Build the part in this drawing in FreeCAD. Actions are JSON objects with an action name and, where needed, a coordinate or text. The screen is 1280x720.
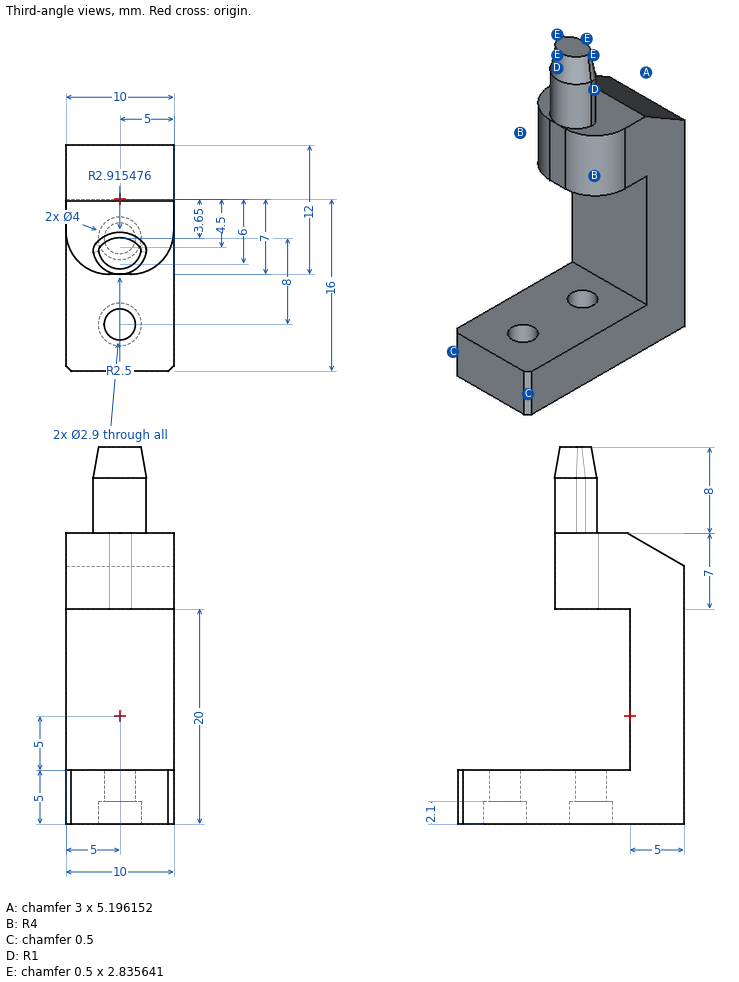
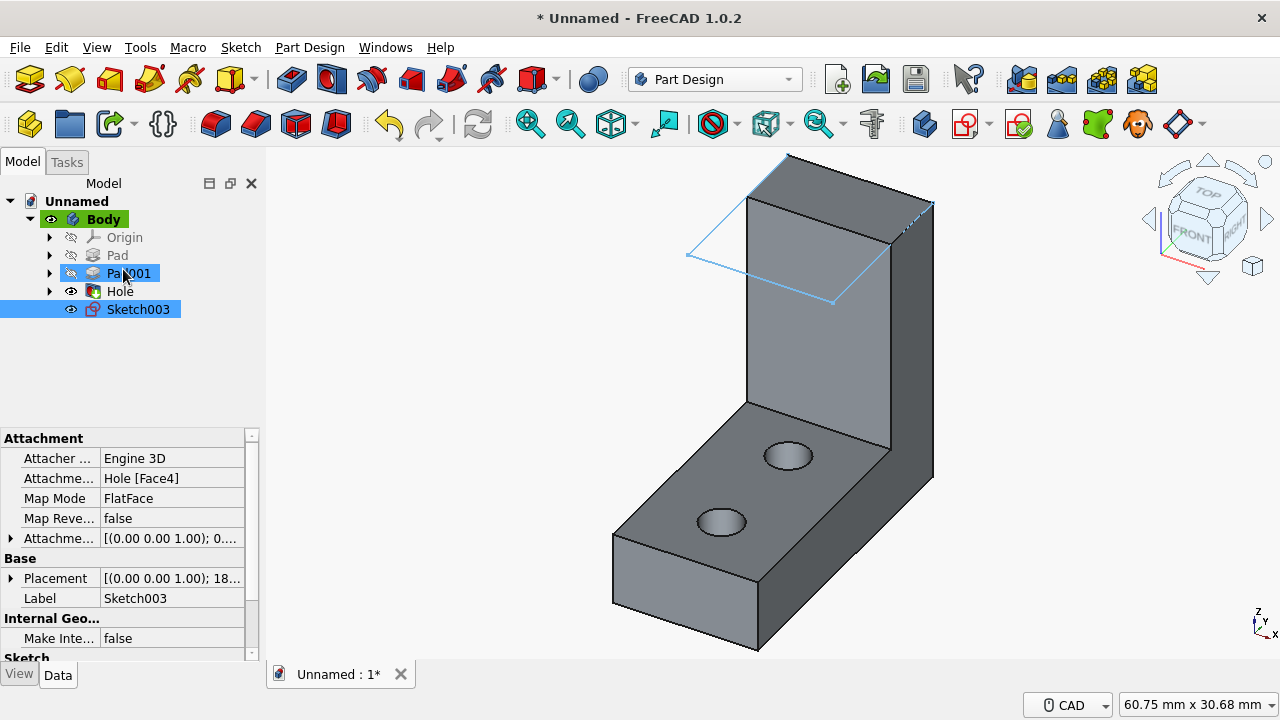
{"action": "left_click", "coordinate": [30, 80]}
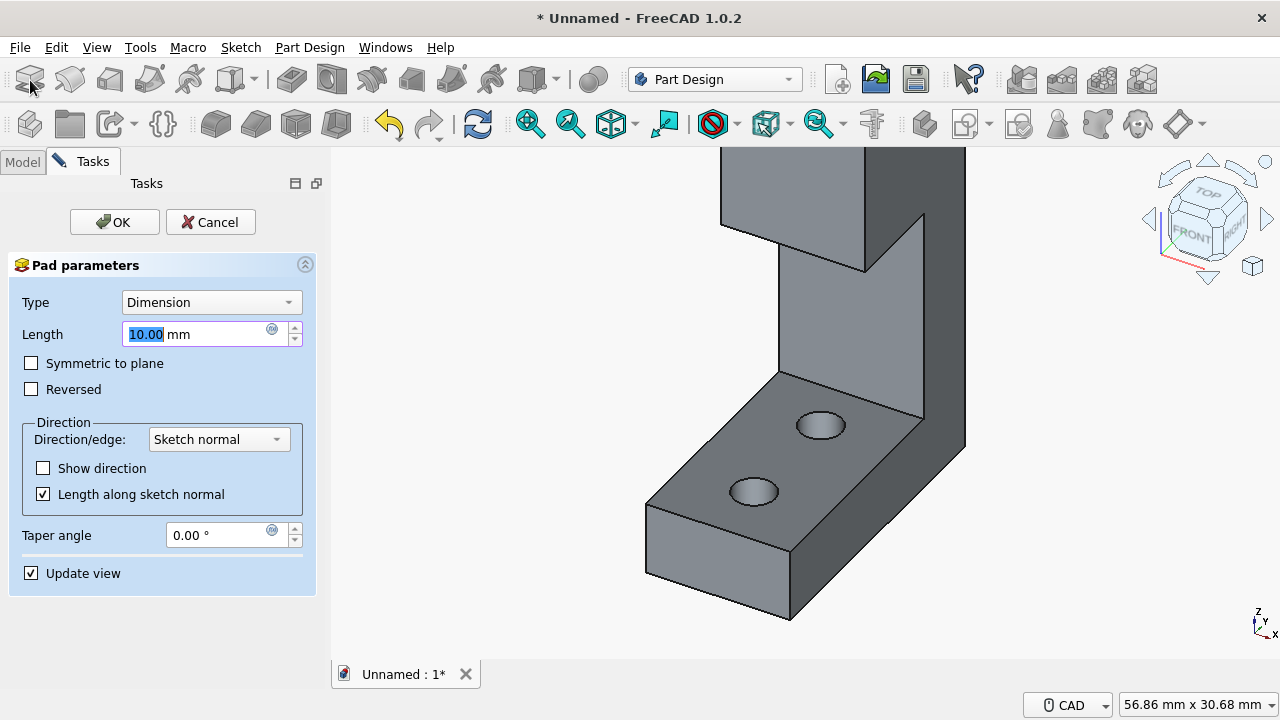
{"action": "type", "text": "7"}
{"action": "key", "text": "Tab"}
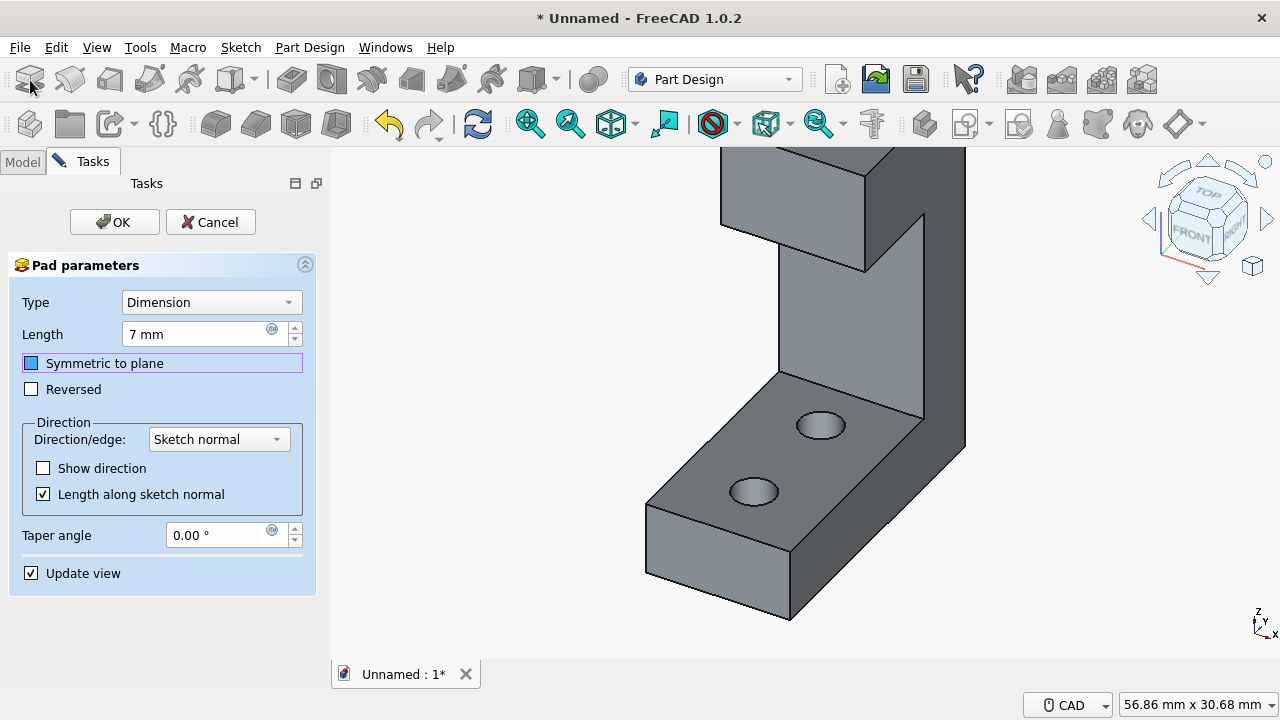
{"action": "left_click", "coordinate": [115, 222]}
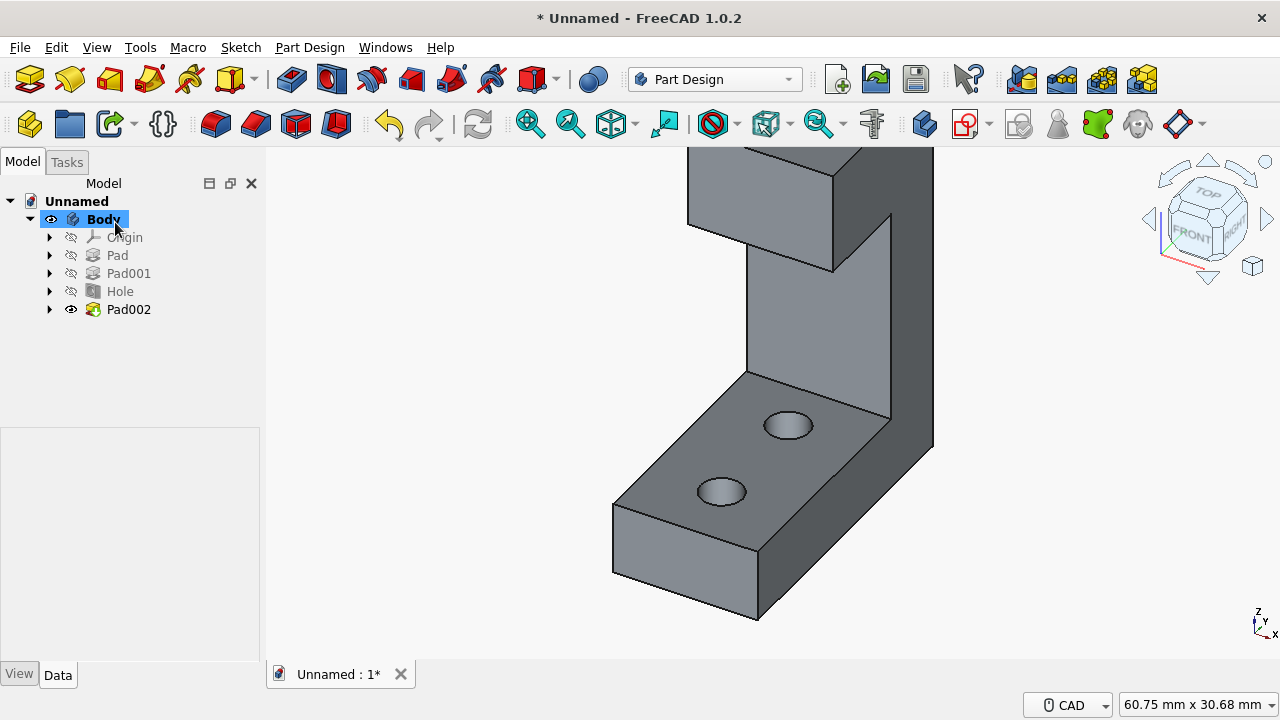
{"action": "left_click", "coordinate": [532, 124]}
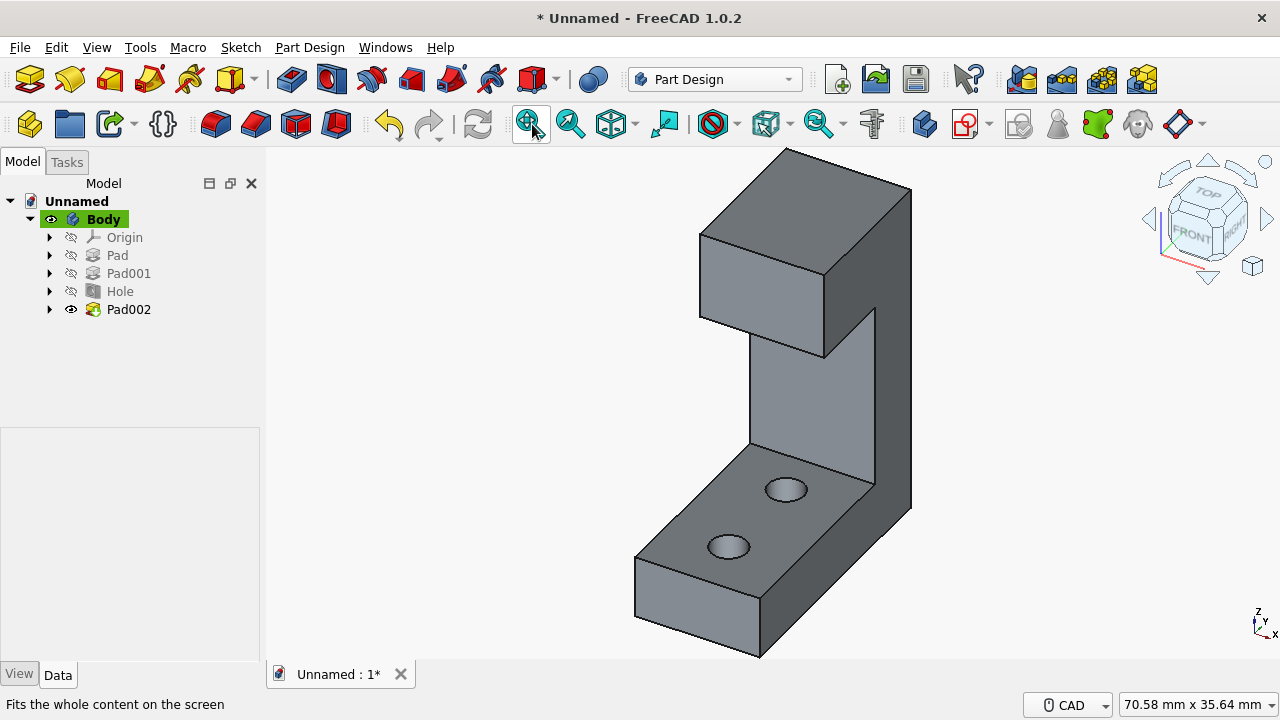
{"action": "key", "text": "0"}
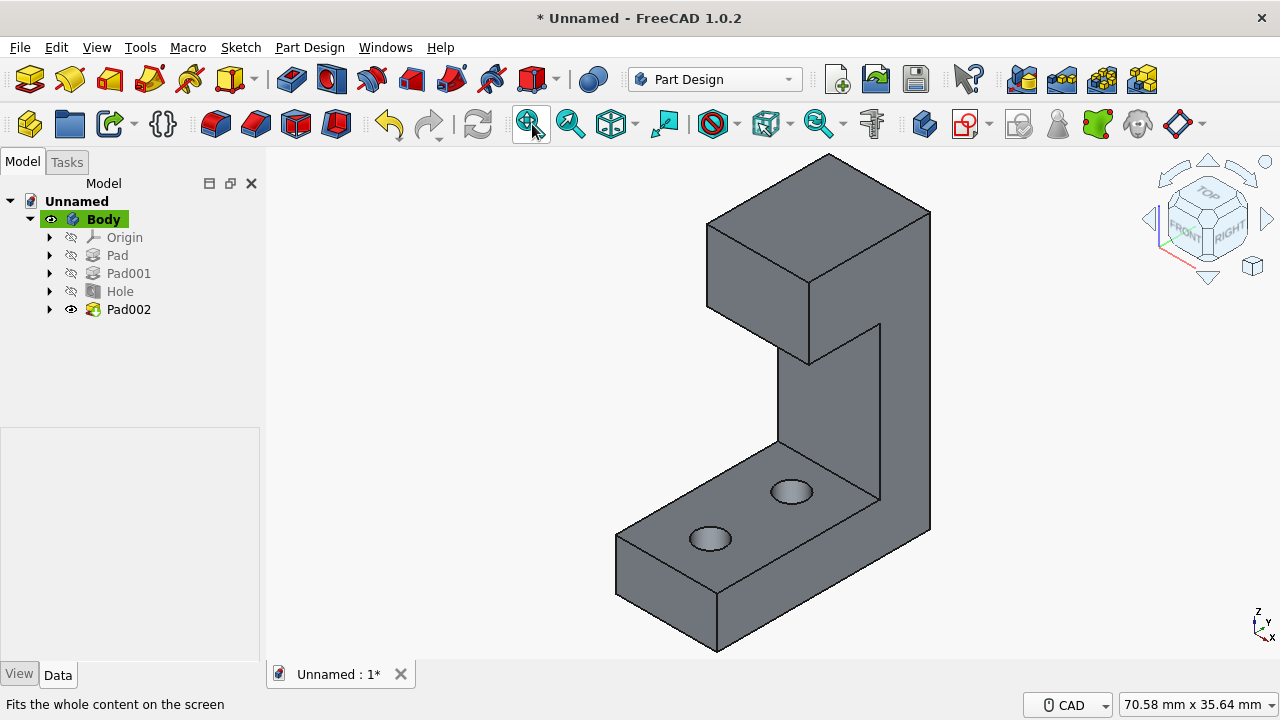
{"action": "key", "text": "2"}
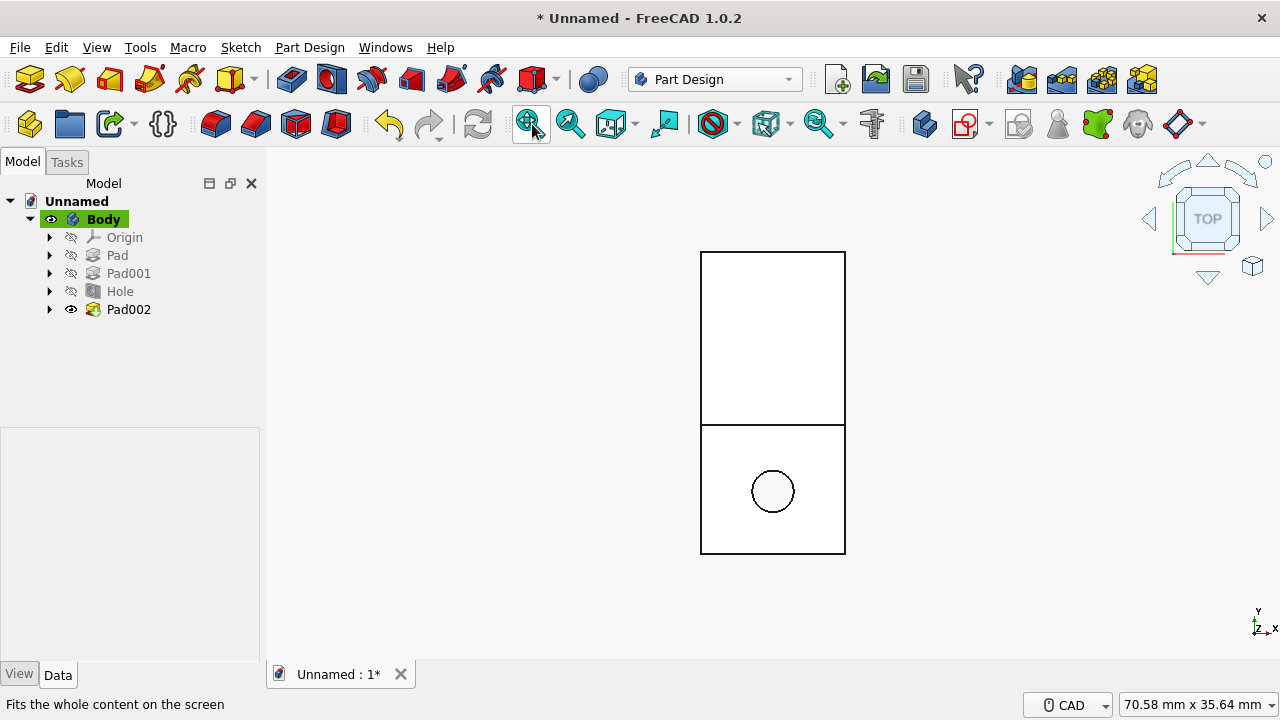
{"action": "left_click", "coordinate": [773, 251]}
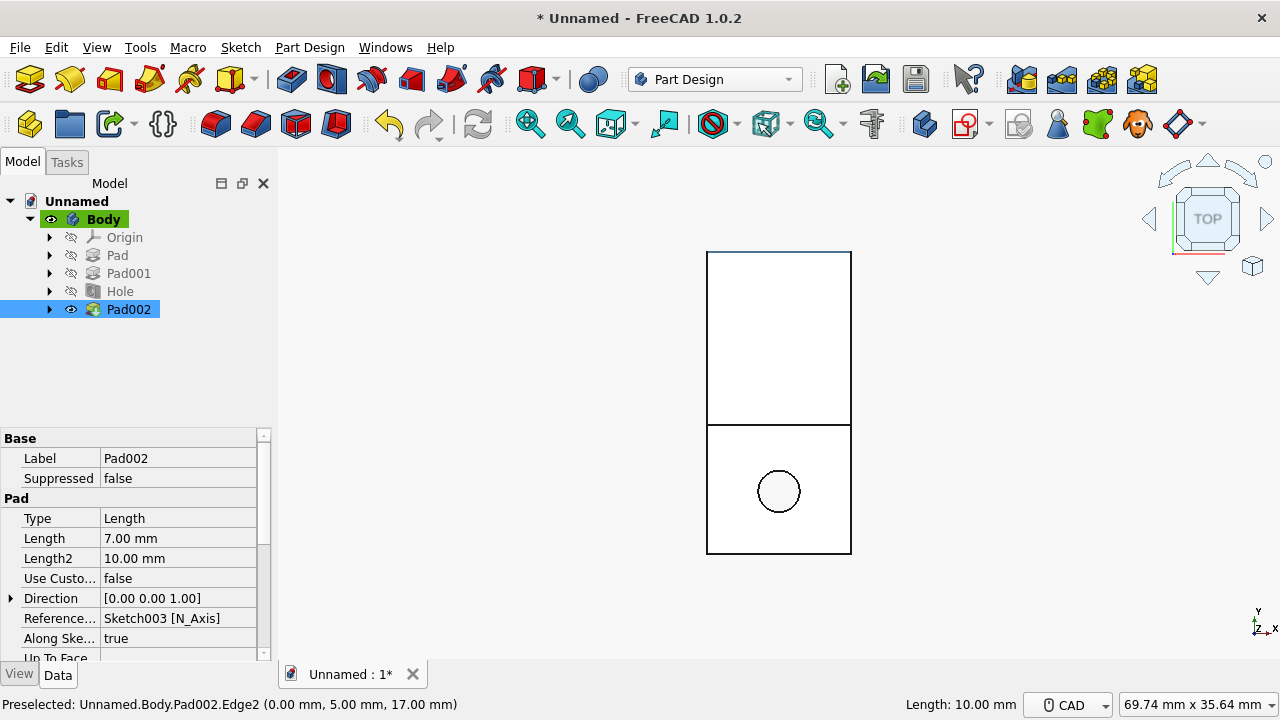
{"action": "left_click", "coordinate": [256, 124]}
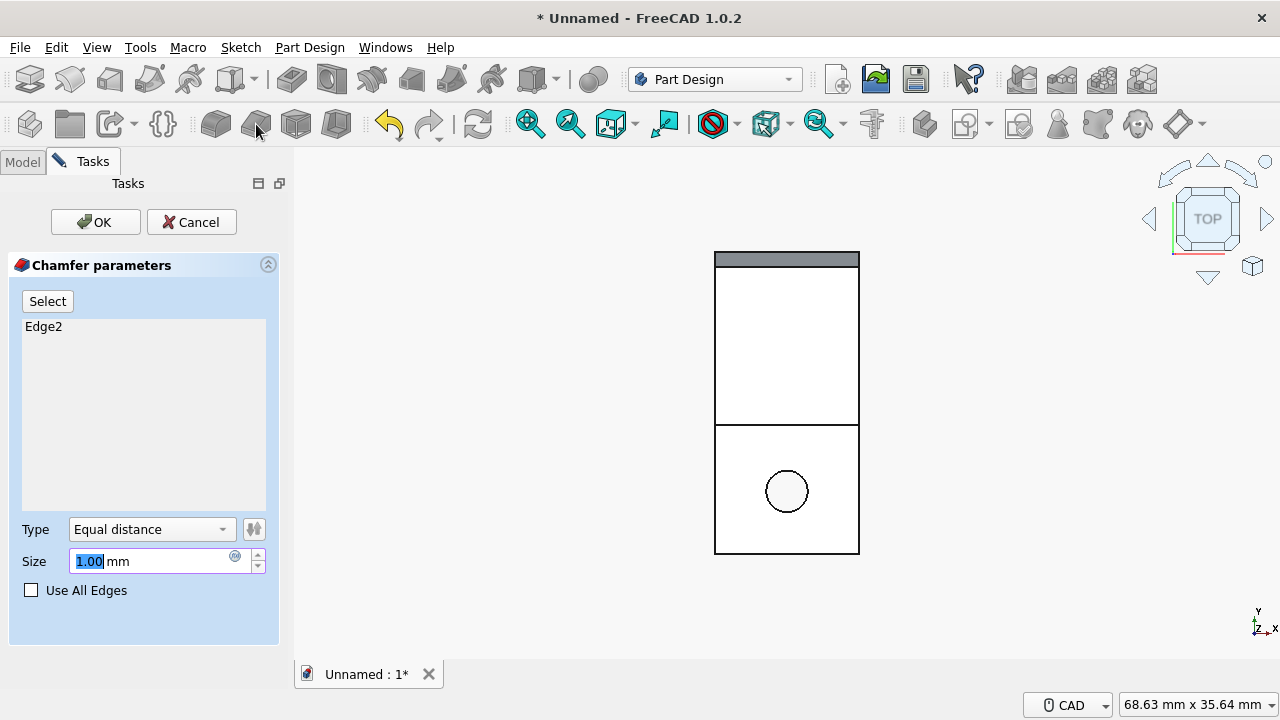
{"action": "type", "text": "3"}
{"action": "key", "text": "Tab"}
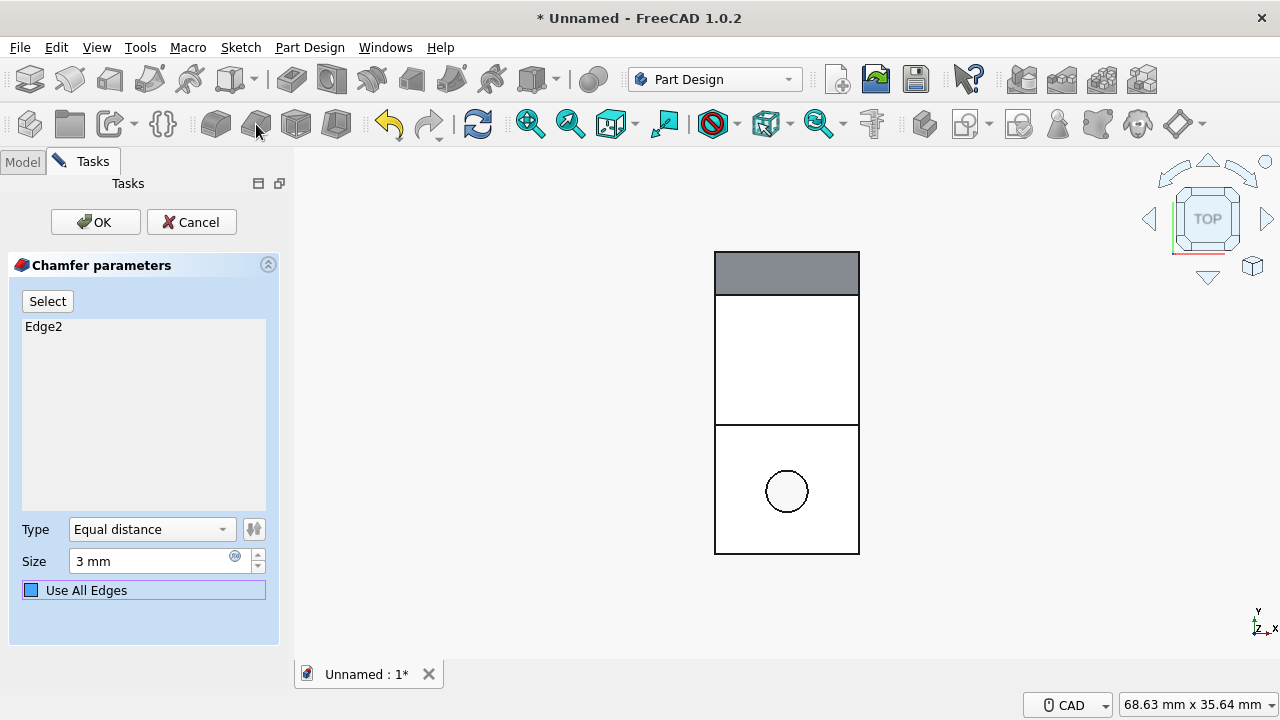
{"action": "left_click", "coordinate": [153, 530]}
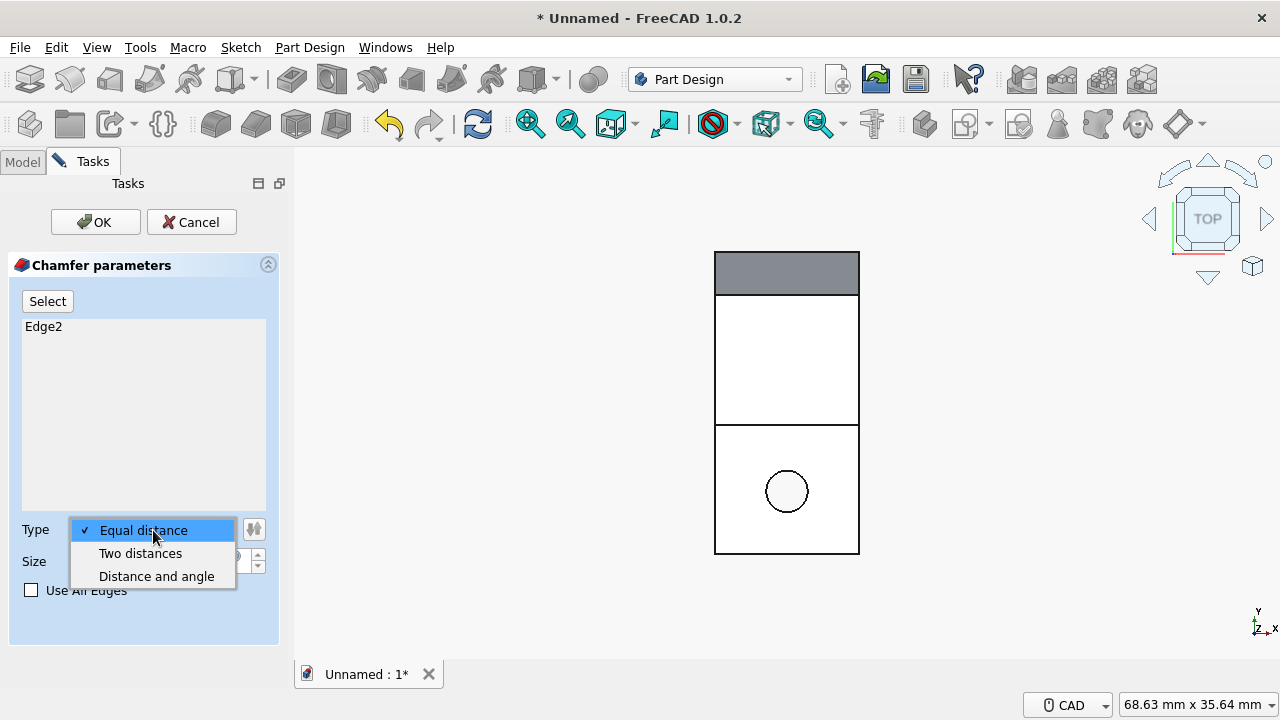
{"action": "left_click", "coordinate": [152, 554]}